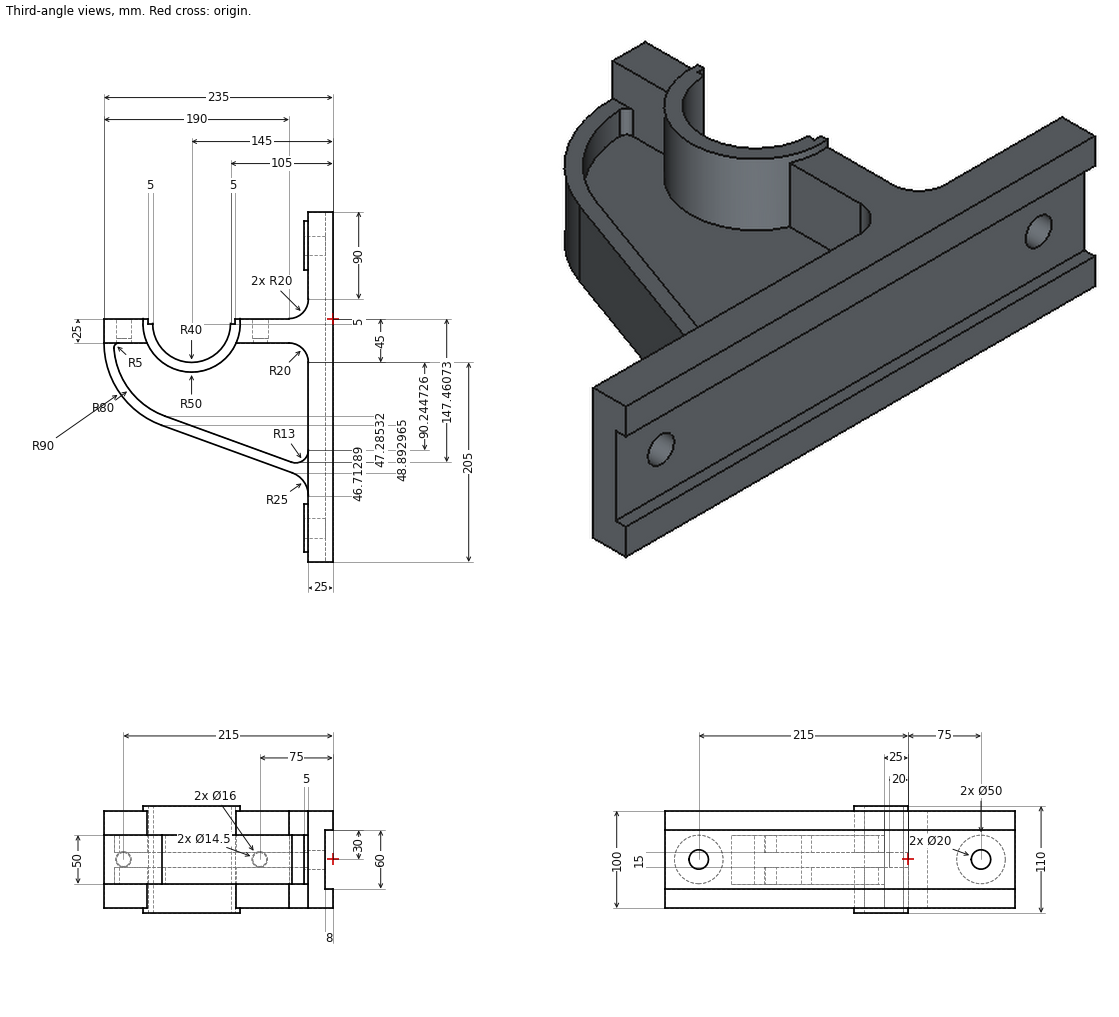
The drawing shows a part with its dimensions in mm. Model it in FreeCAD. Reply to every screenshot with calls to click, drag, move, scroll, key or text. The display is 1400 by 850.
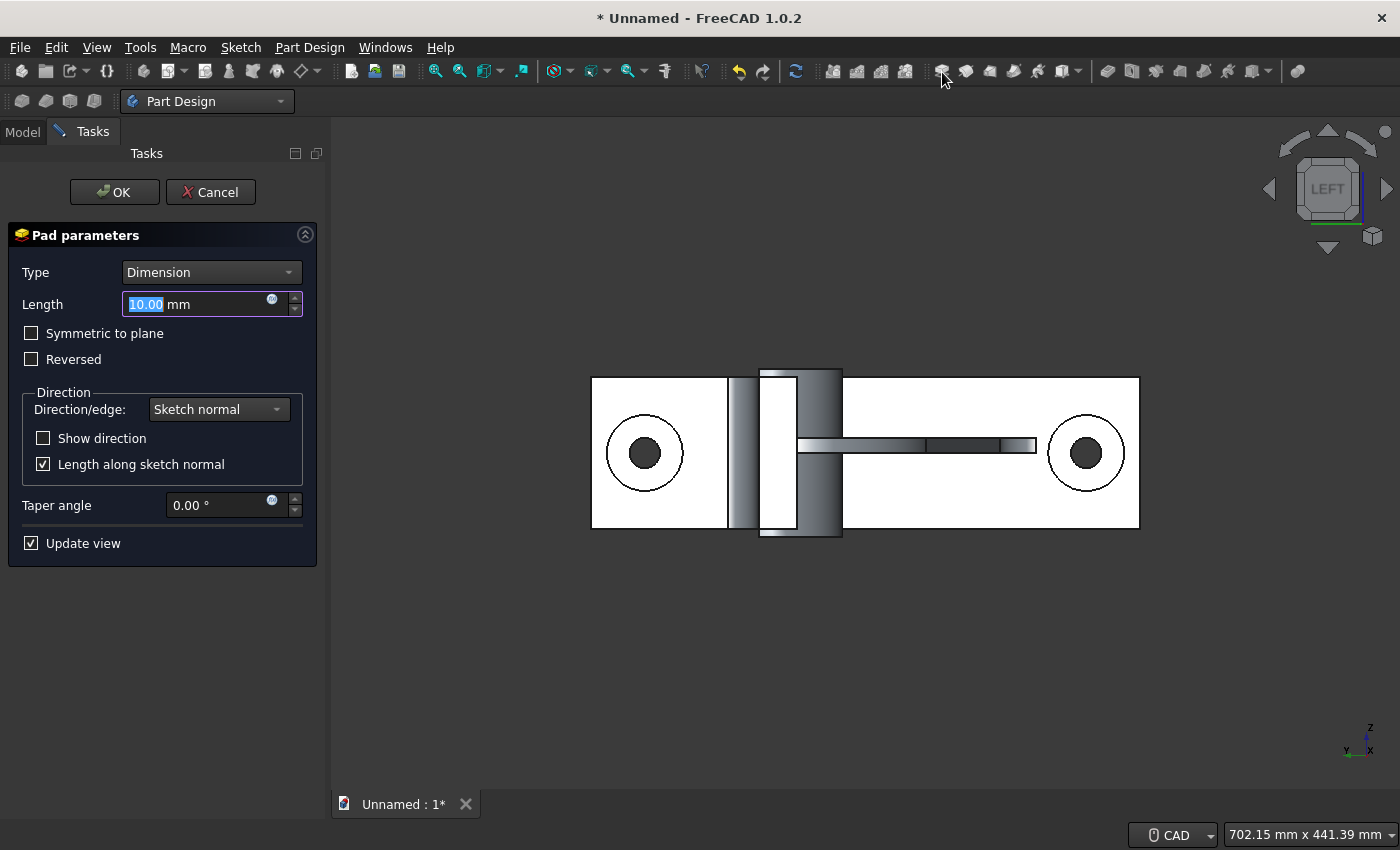
text(50)
key(Tab)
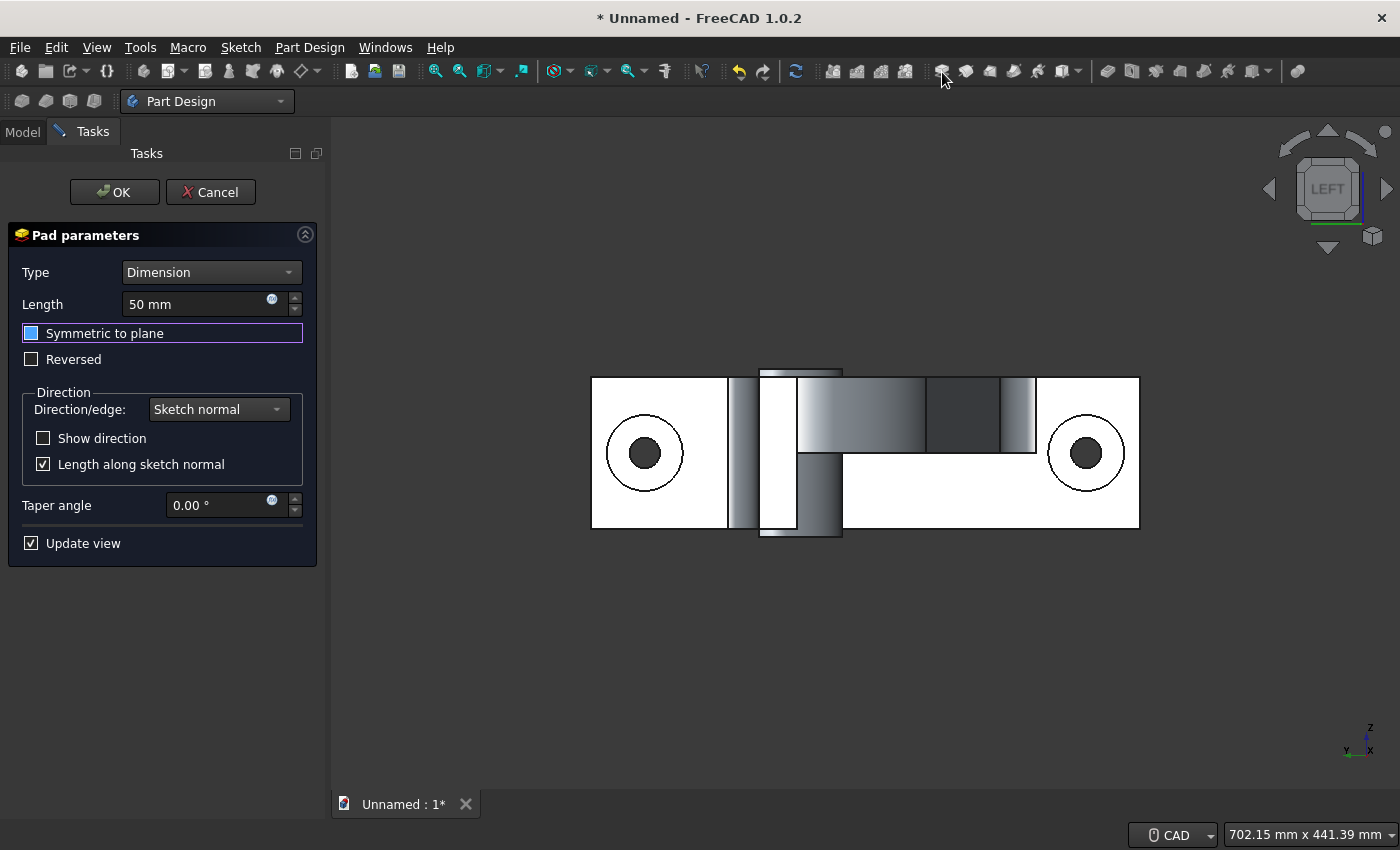
click(30, 333)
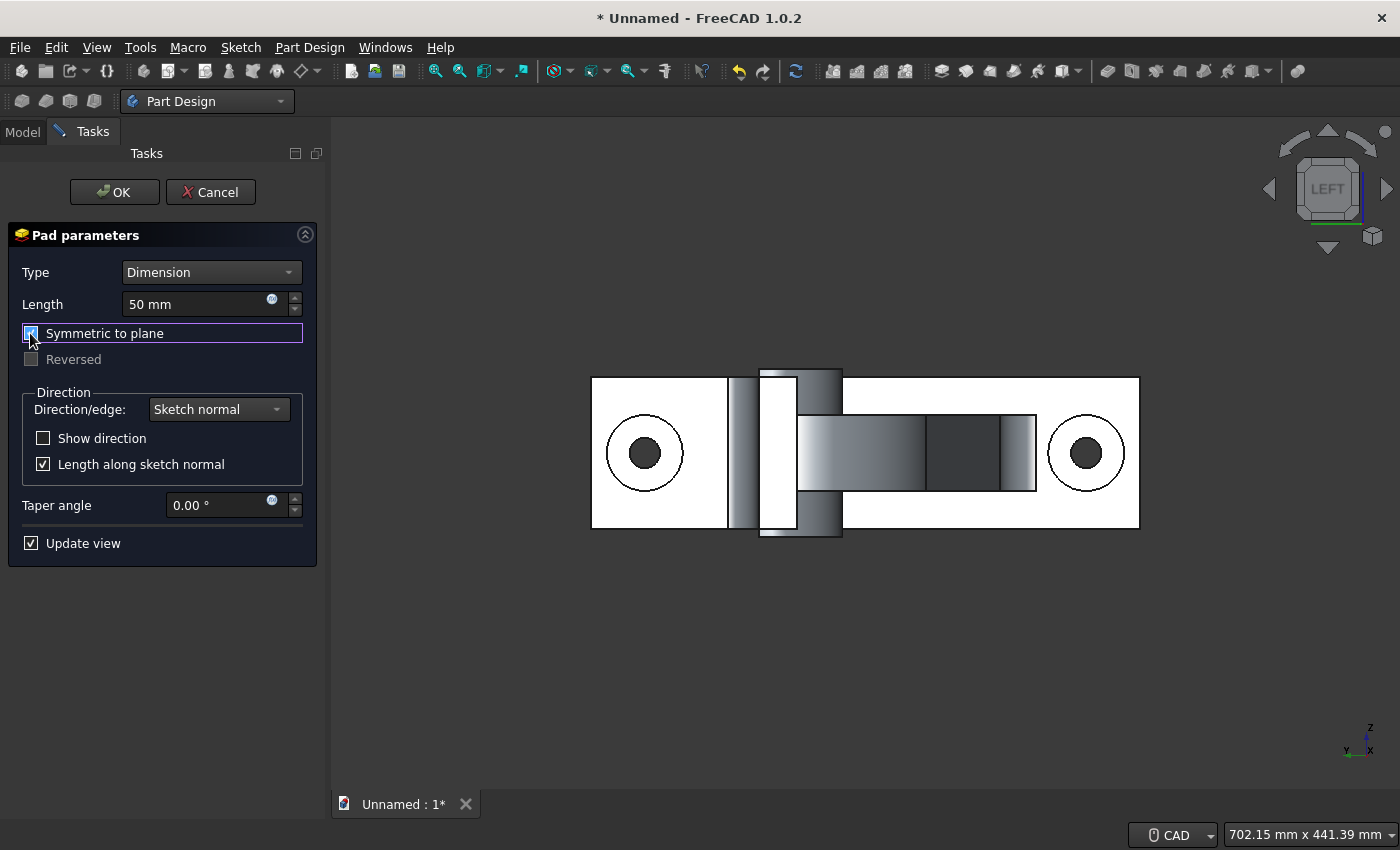
click(115, 192)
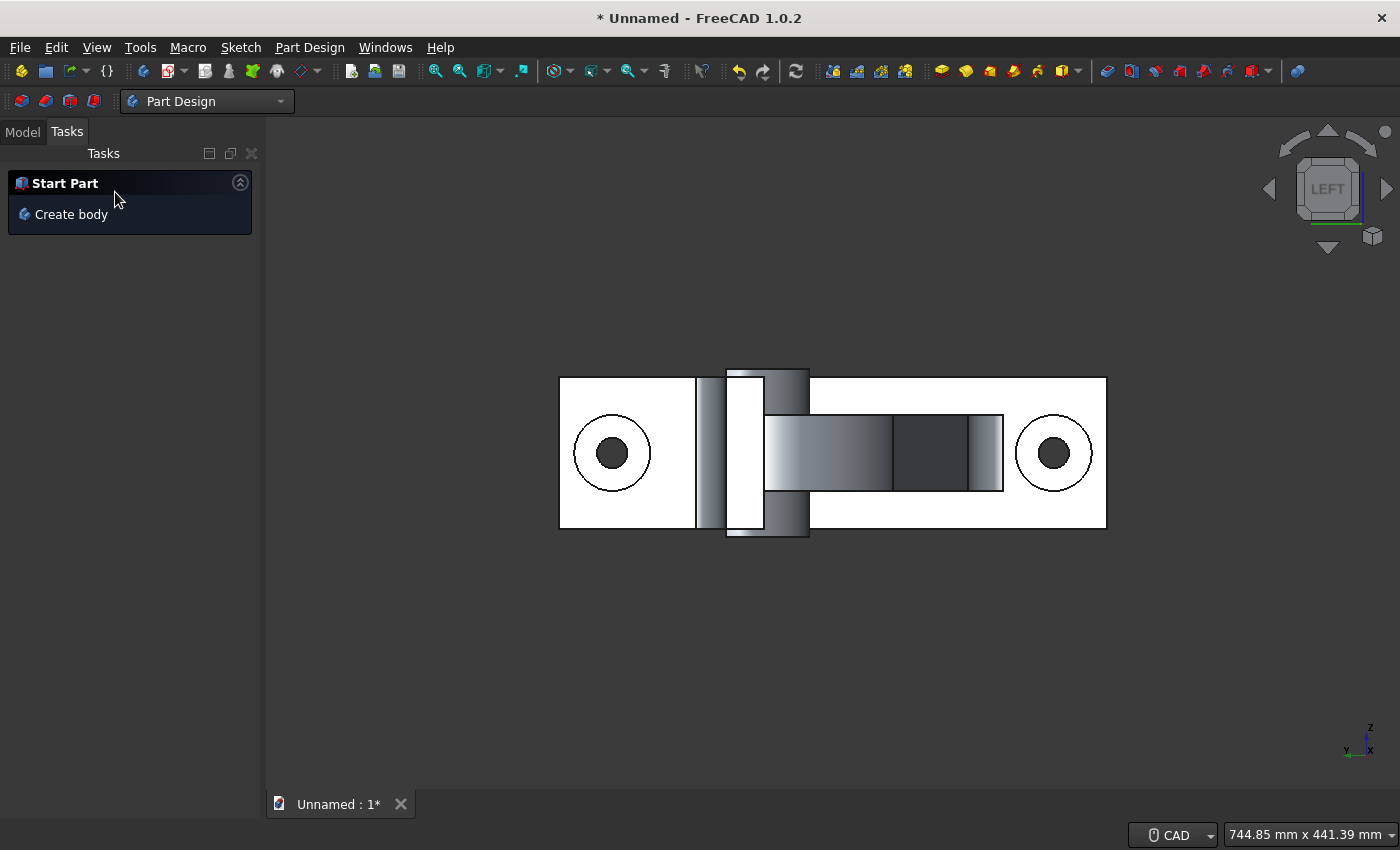
click(168, 72)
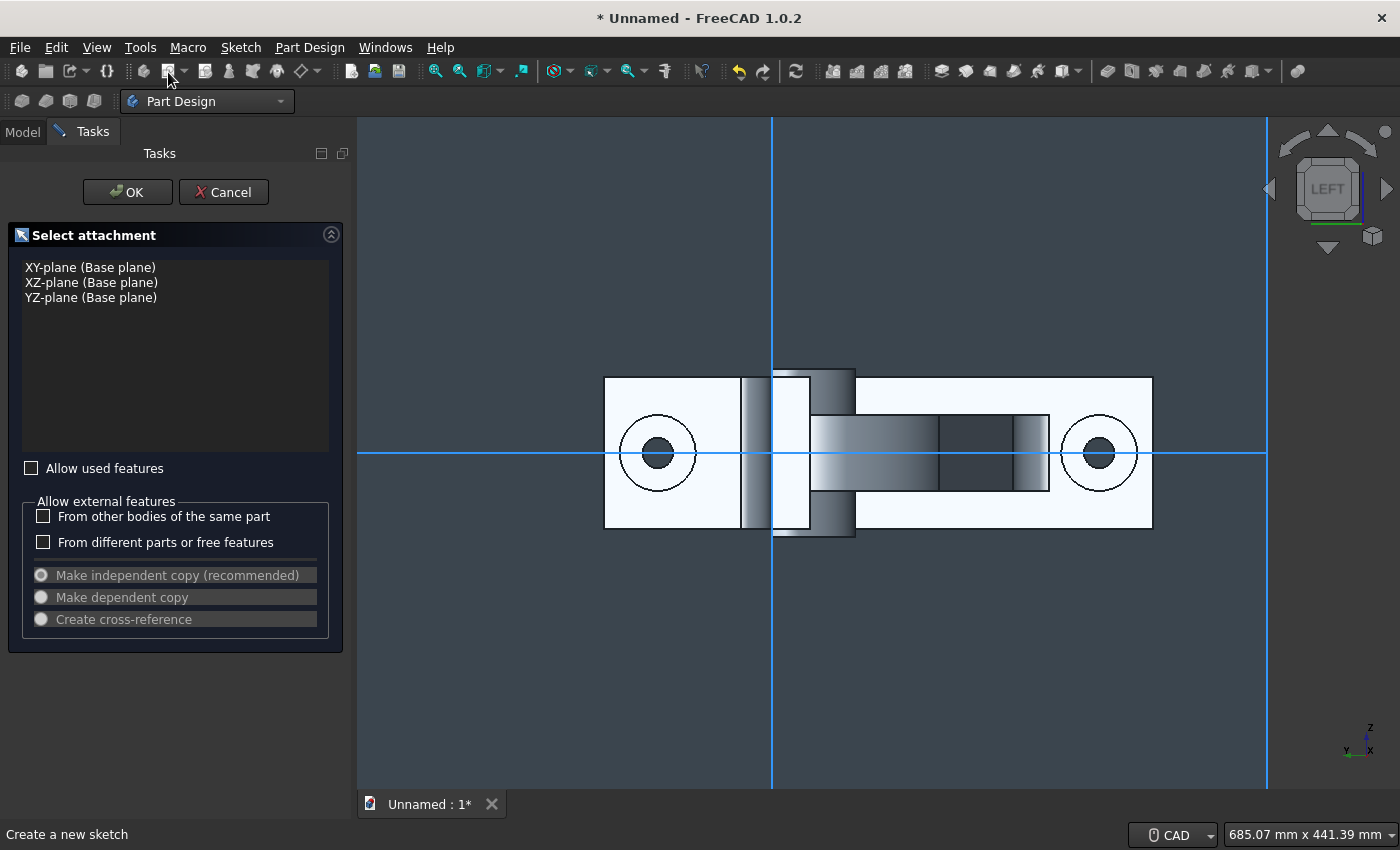
click(82, 268)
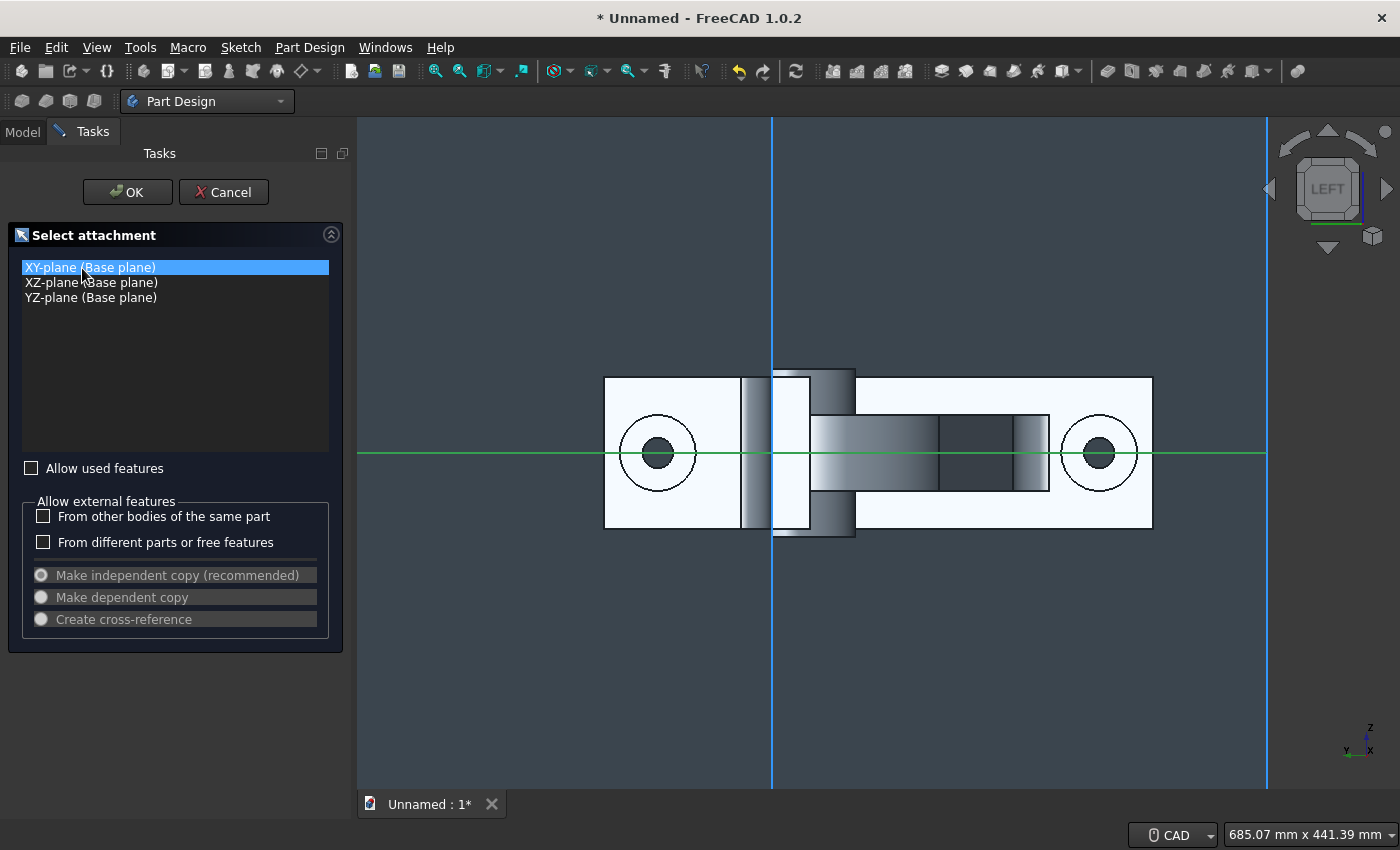
click(128, 192)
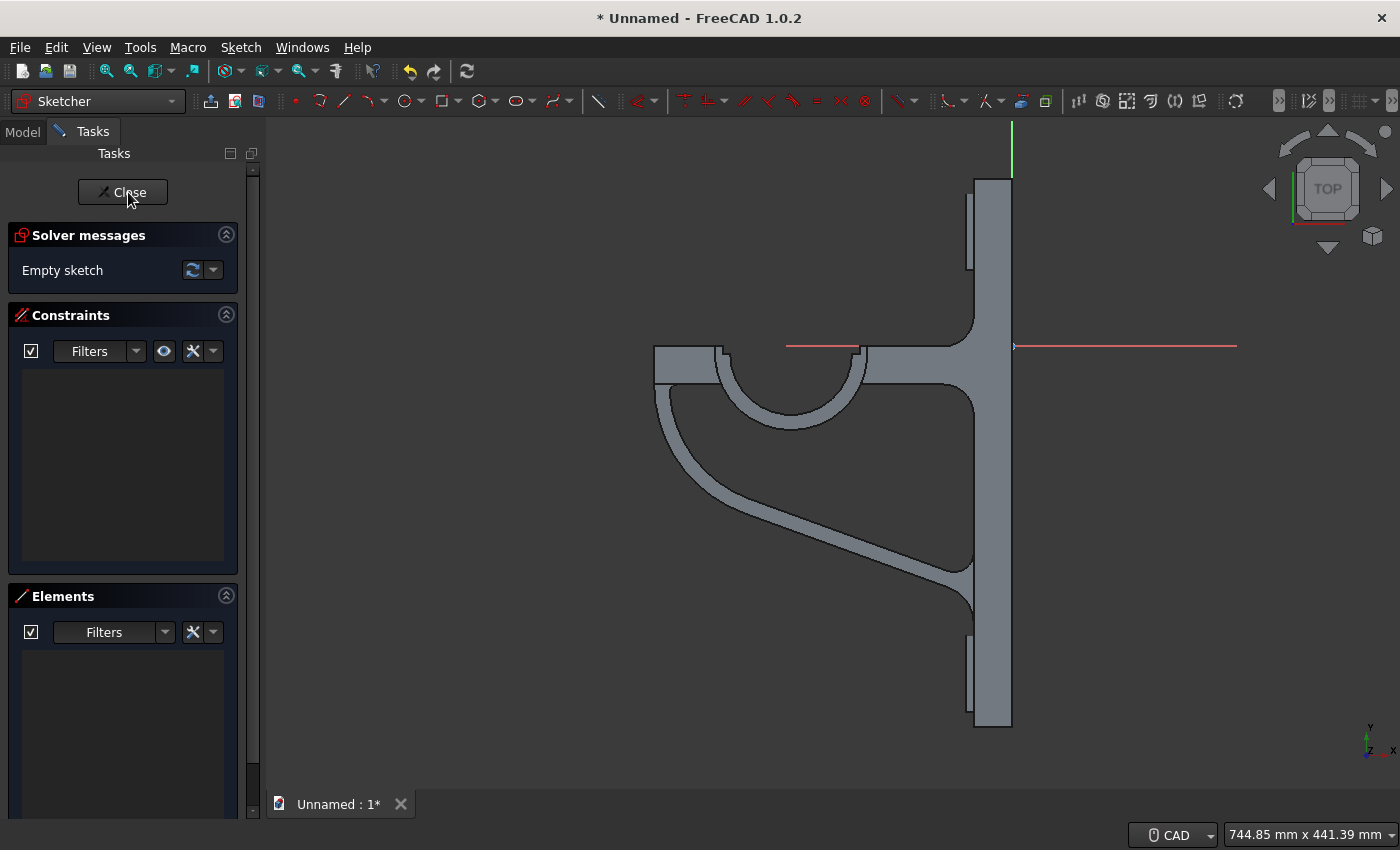
click(260, 102)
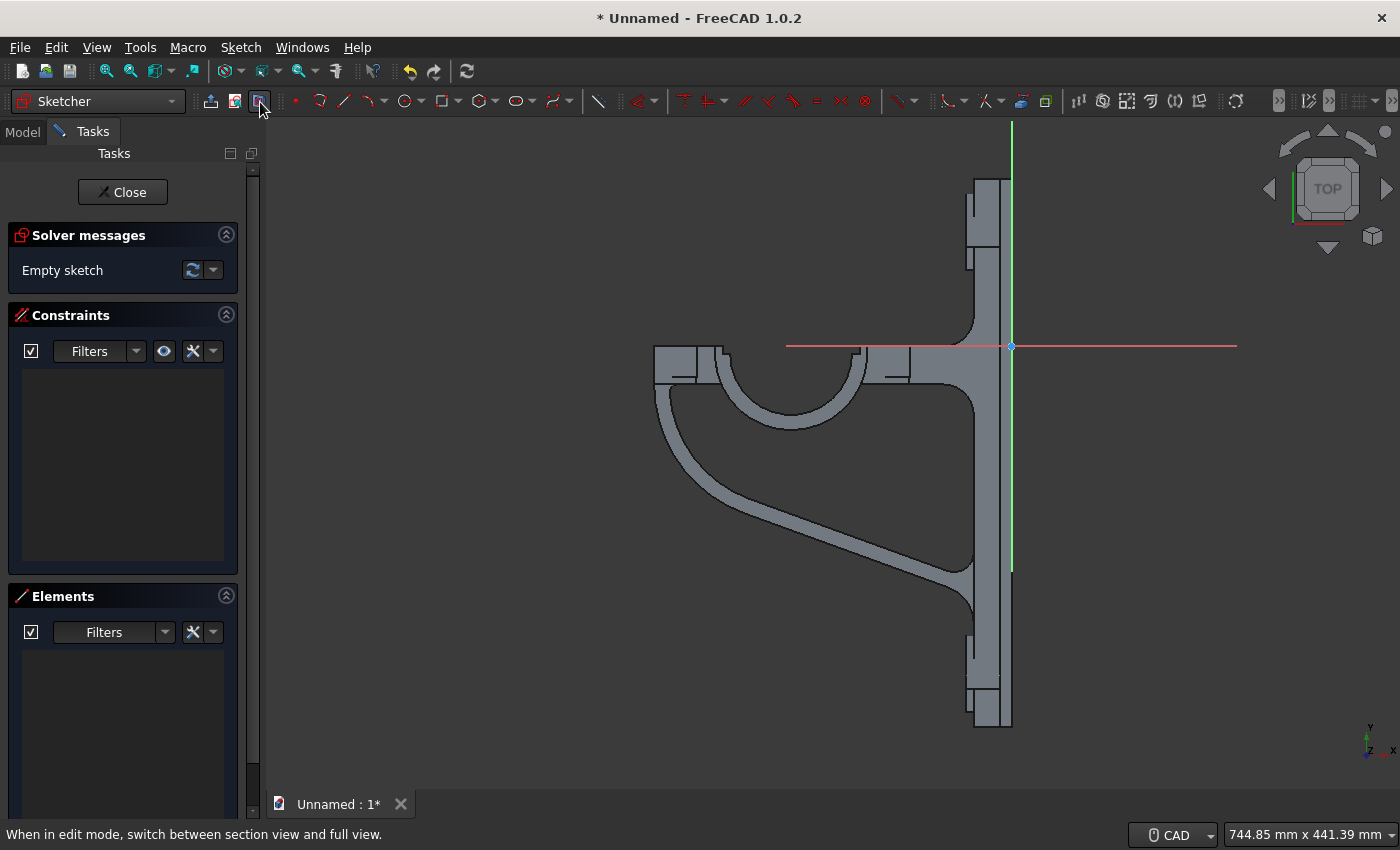
scroll(933, 466, up, 3)